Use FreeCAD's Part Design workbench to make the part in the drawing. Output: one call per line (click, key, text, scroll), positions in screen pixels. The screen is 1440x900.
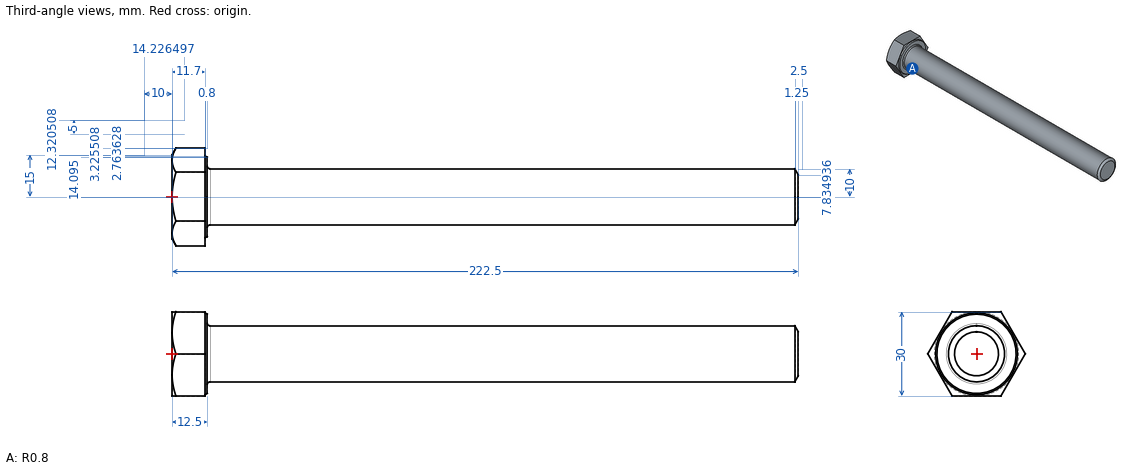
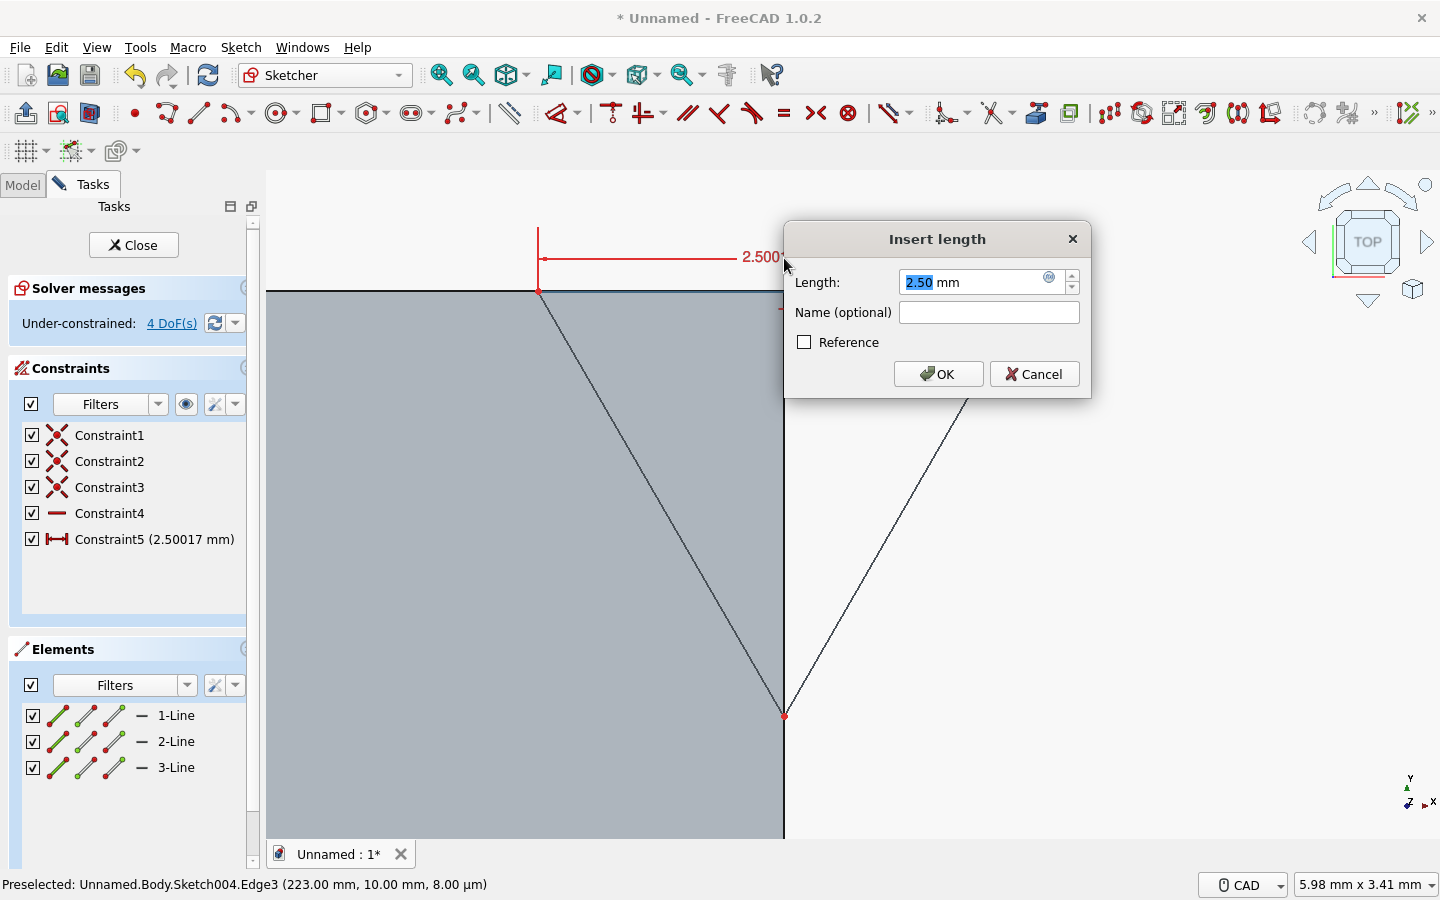
text(2.5)
key(Return)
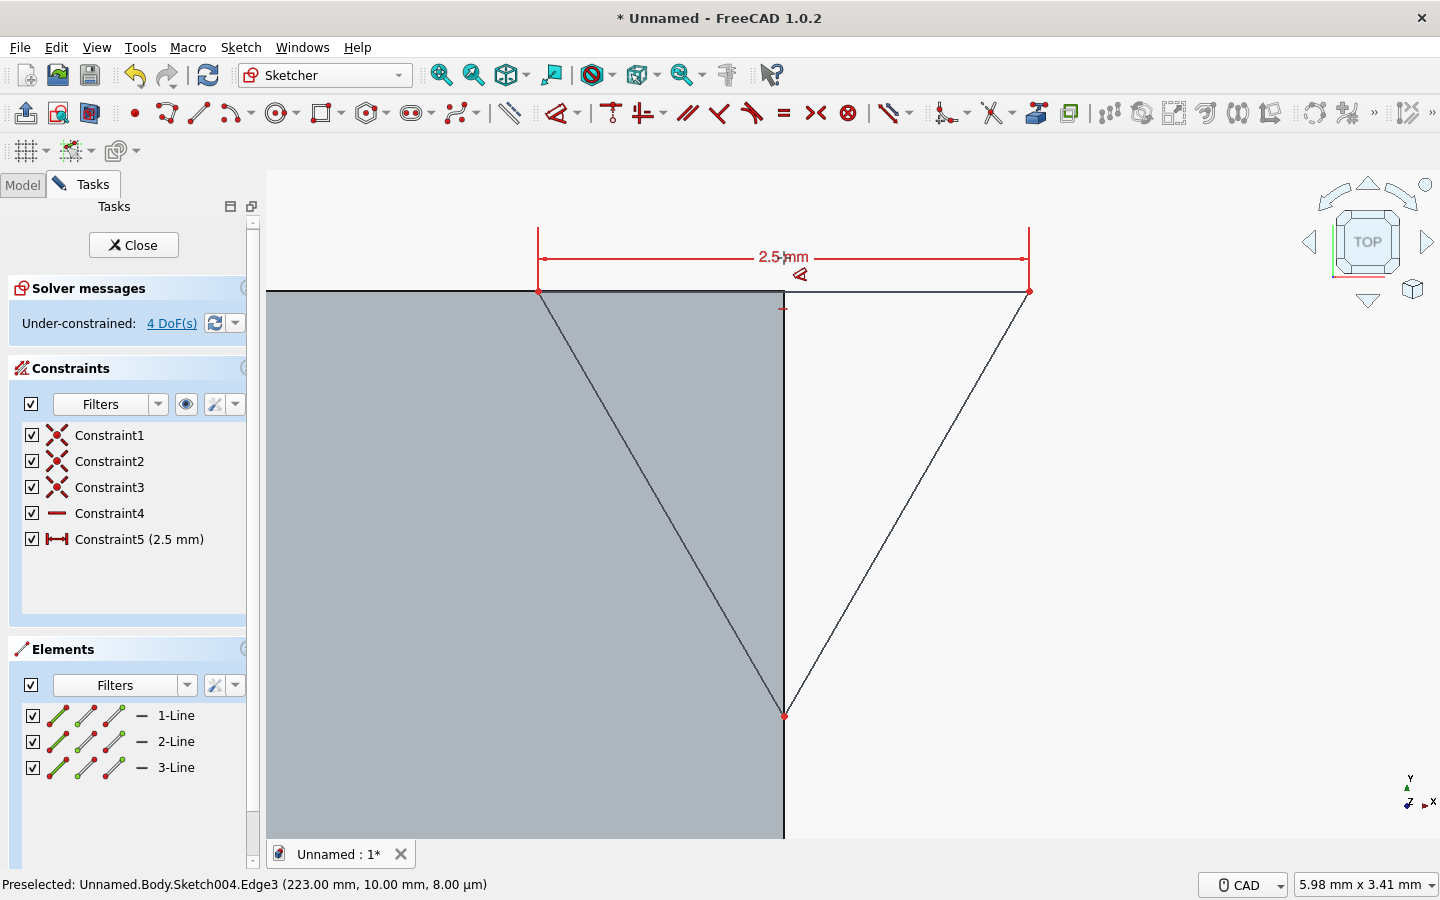
click(538, 292)
click(572, 552)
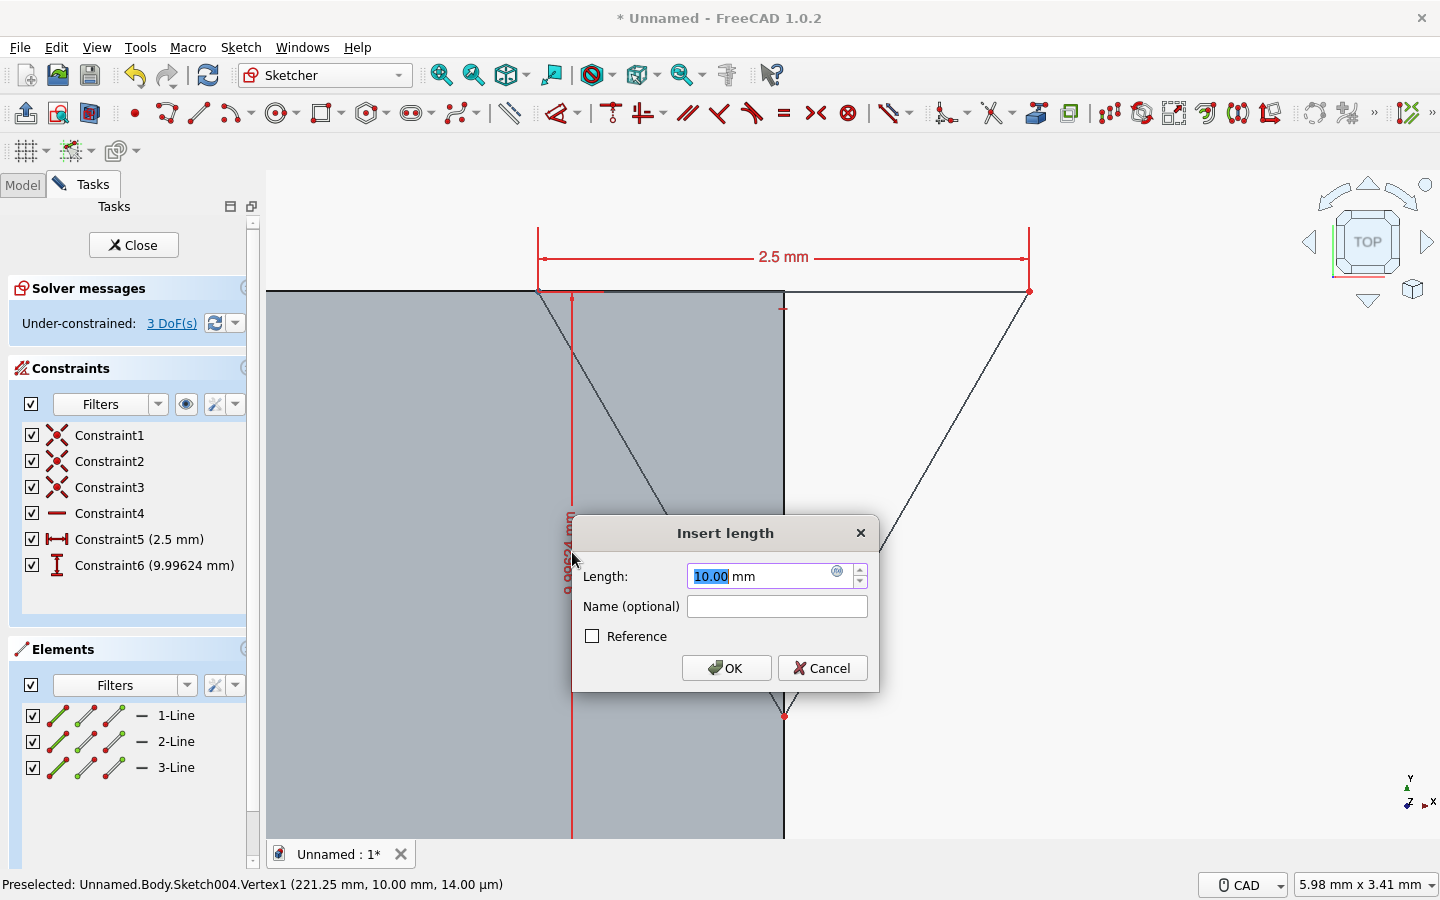
text(10)
key(Return)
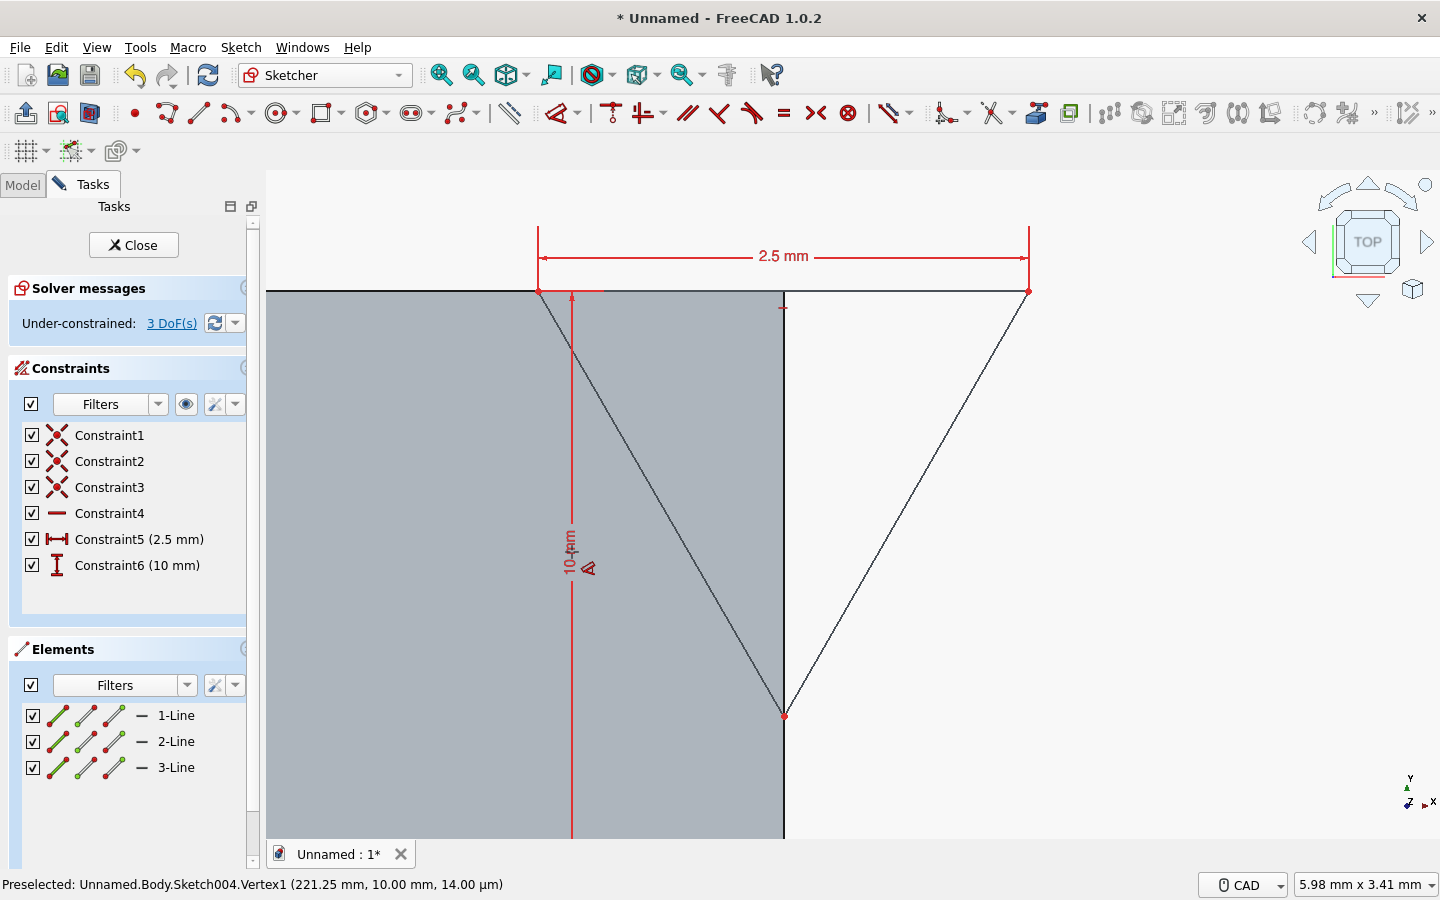
click(612, 419)
click(661, 751)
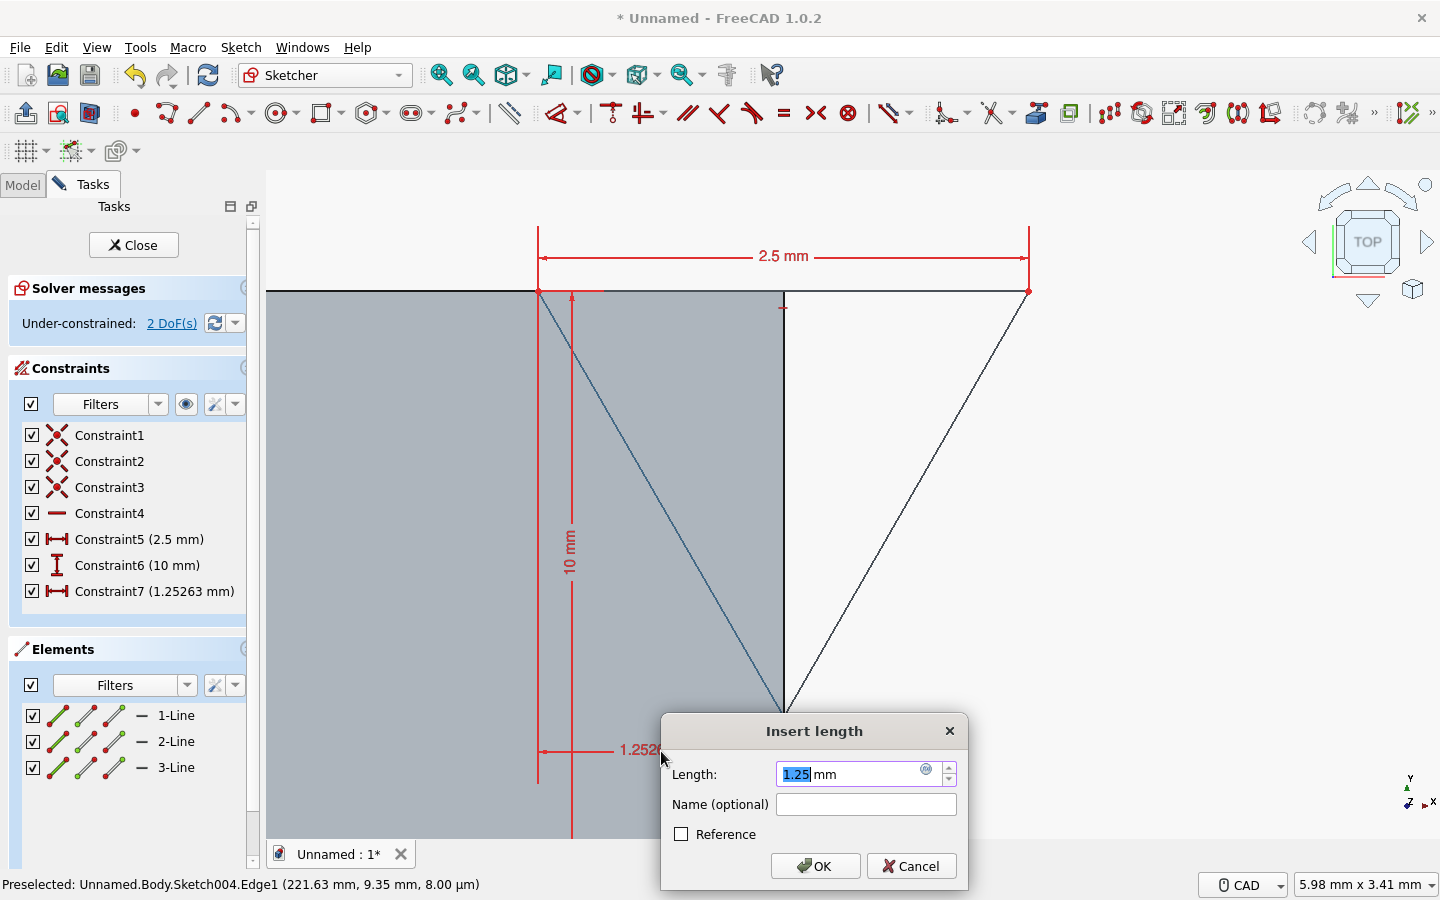
text(1.25)
key(Return)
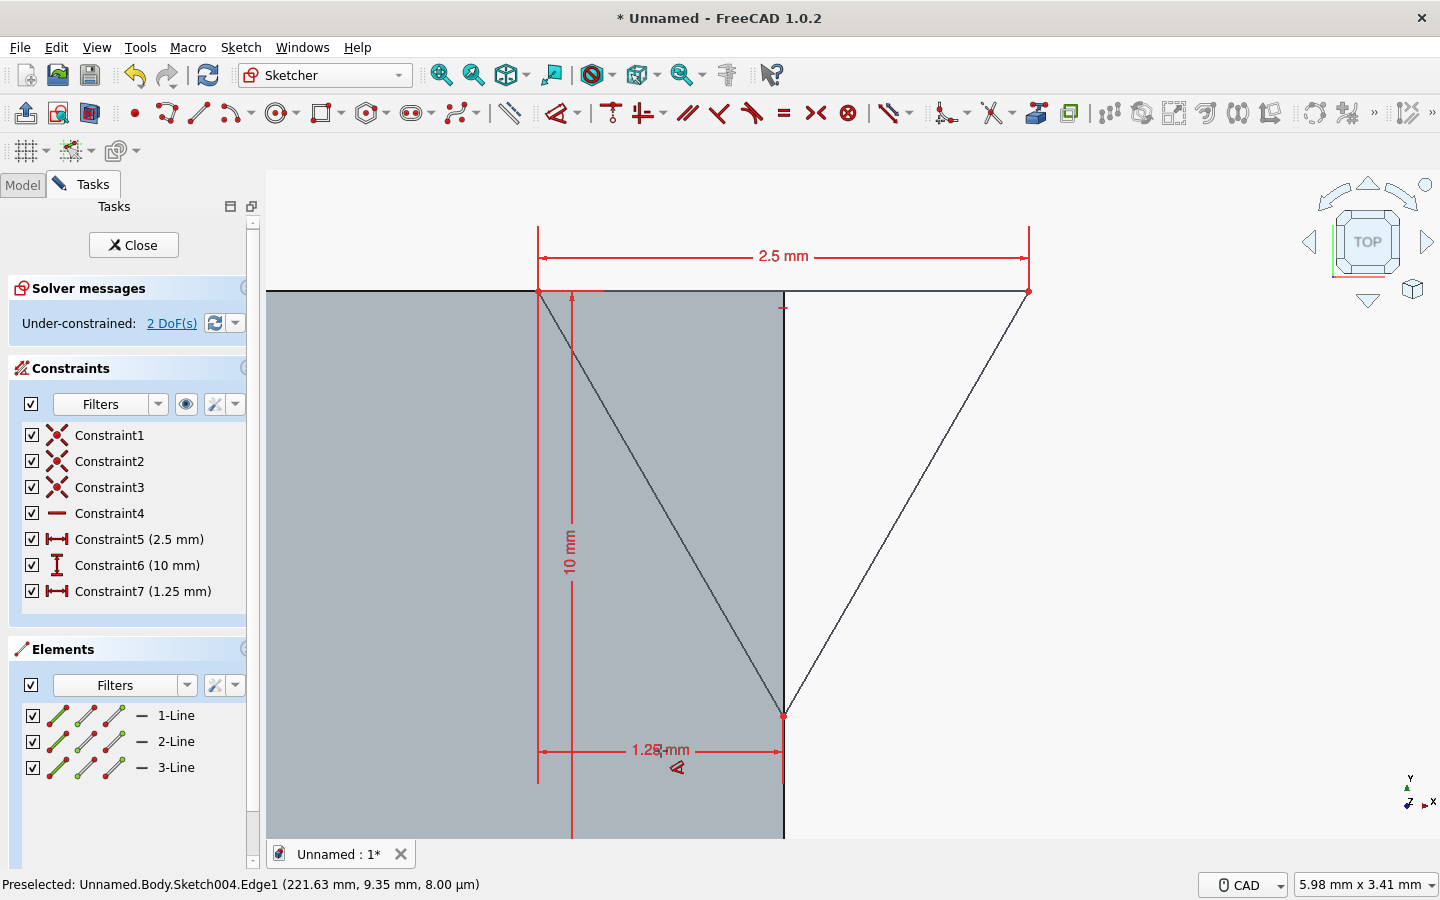
click(783, 717)
click(539, 683)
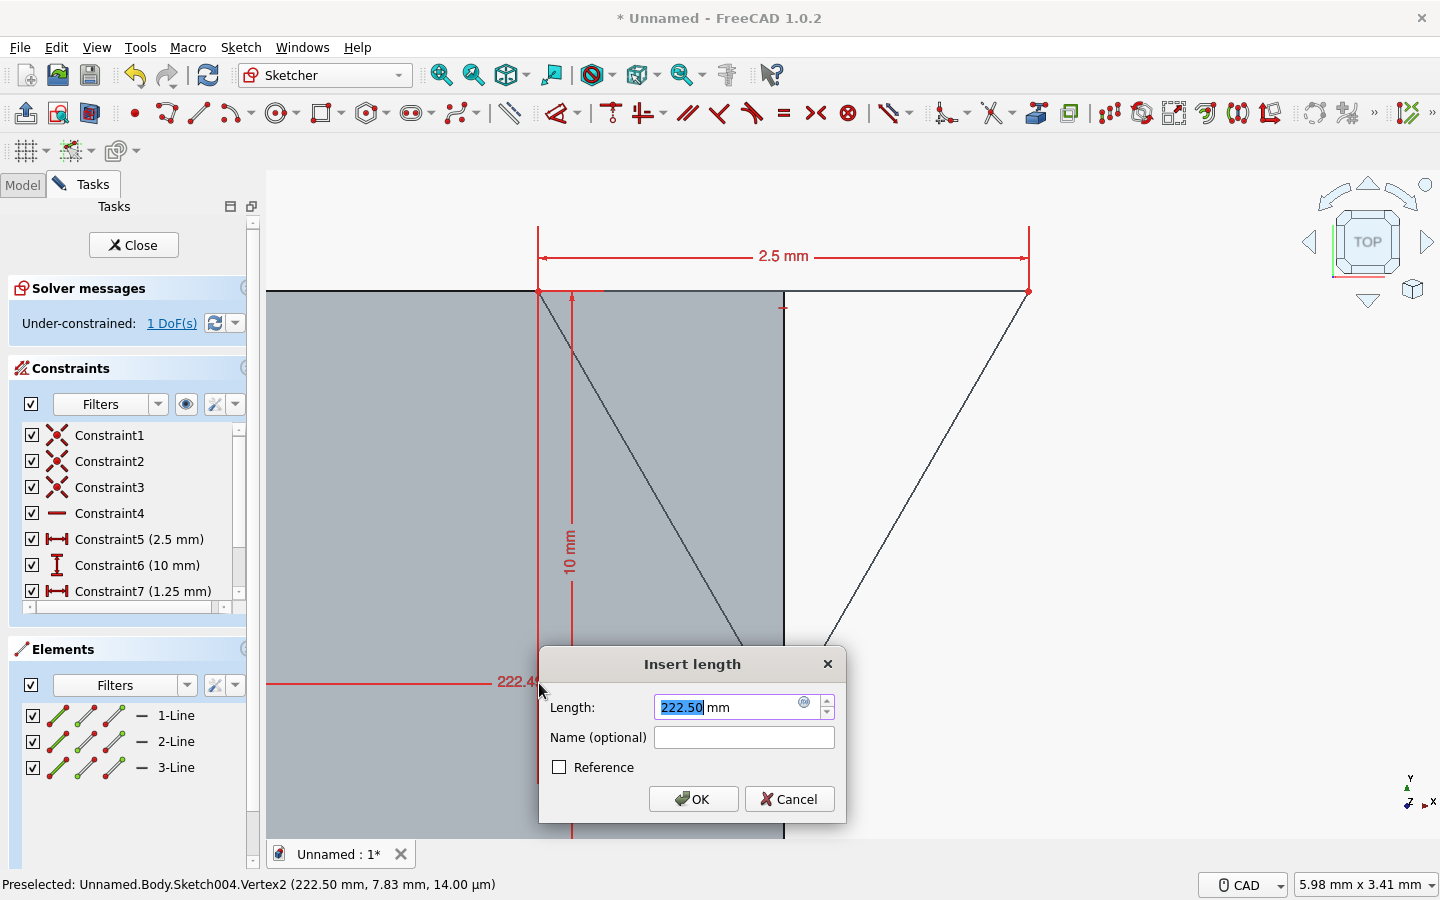
text(222.5)
key(Return)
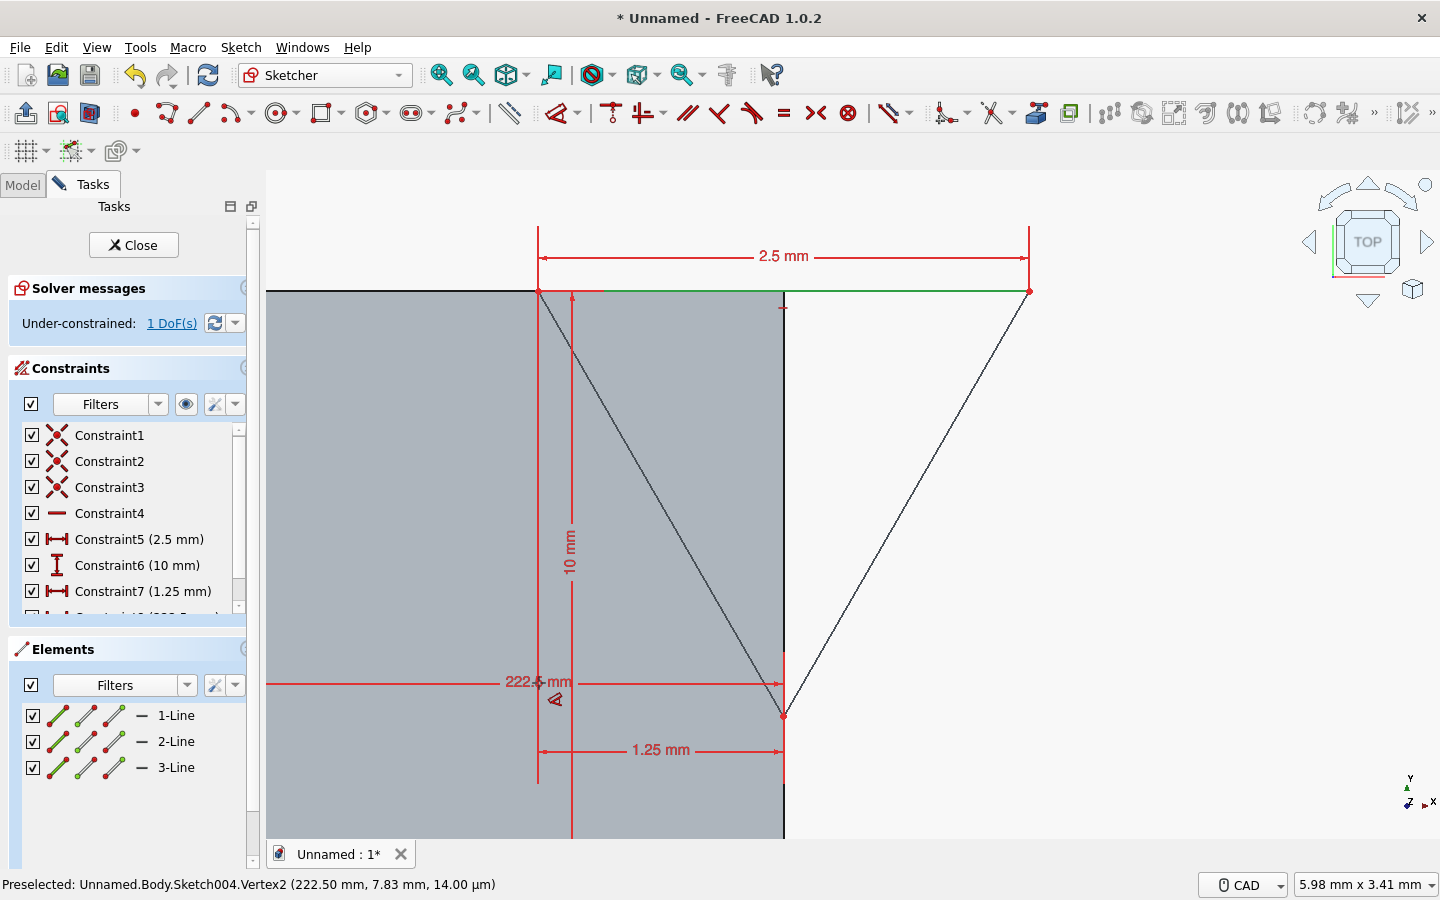
click(784, 717)
click(818, 764)